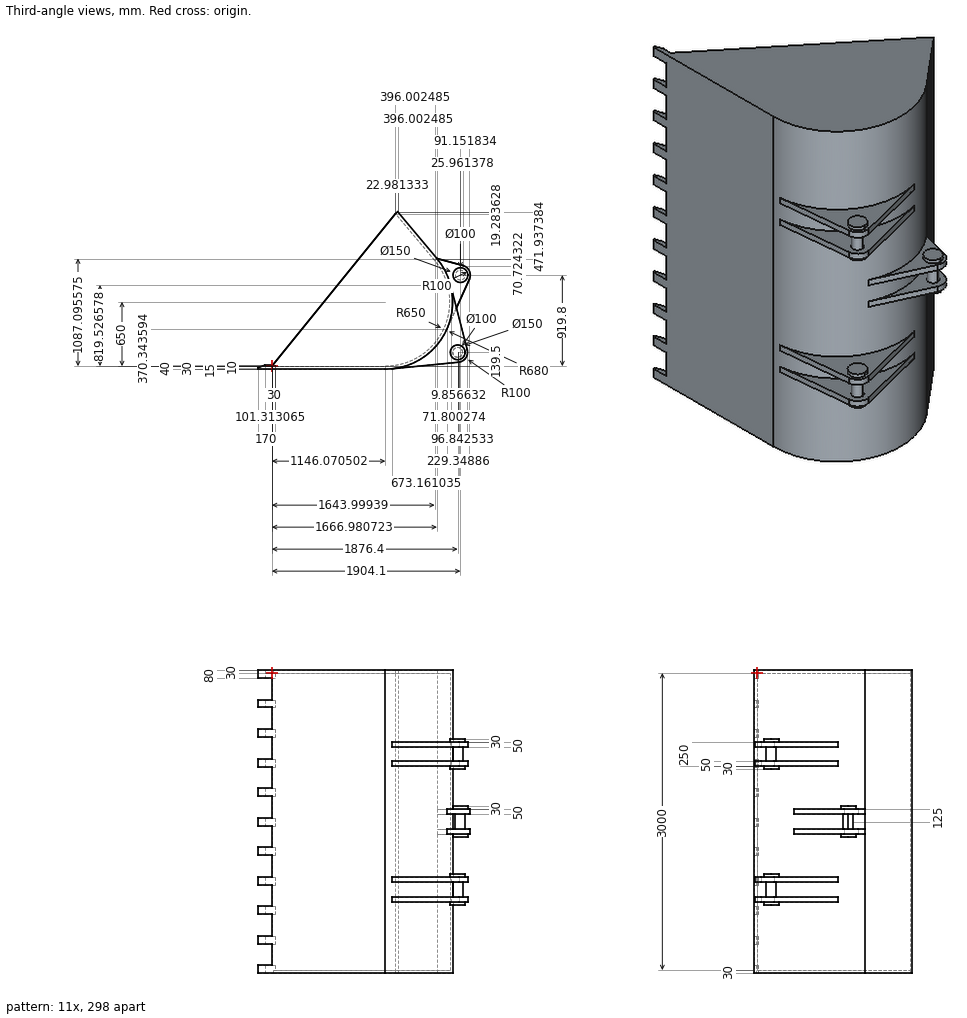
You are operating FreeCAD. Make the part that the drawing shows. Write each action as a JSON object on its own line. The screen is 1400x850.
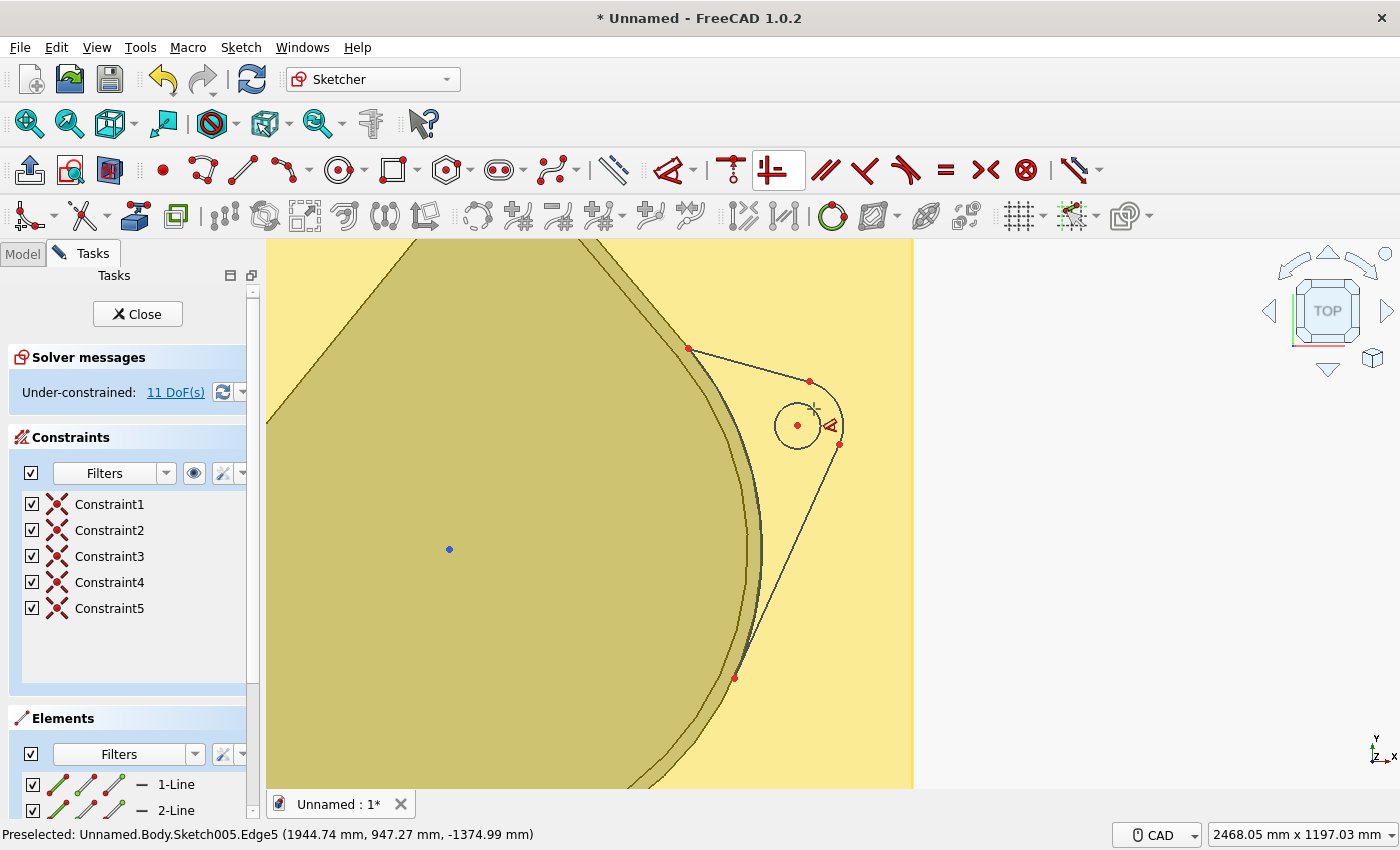
{"action": "left_click", "coordinate": [761, 578]}
{"action": "left_click", "coordinate": [793, 581]}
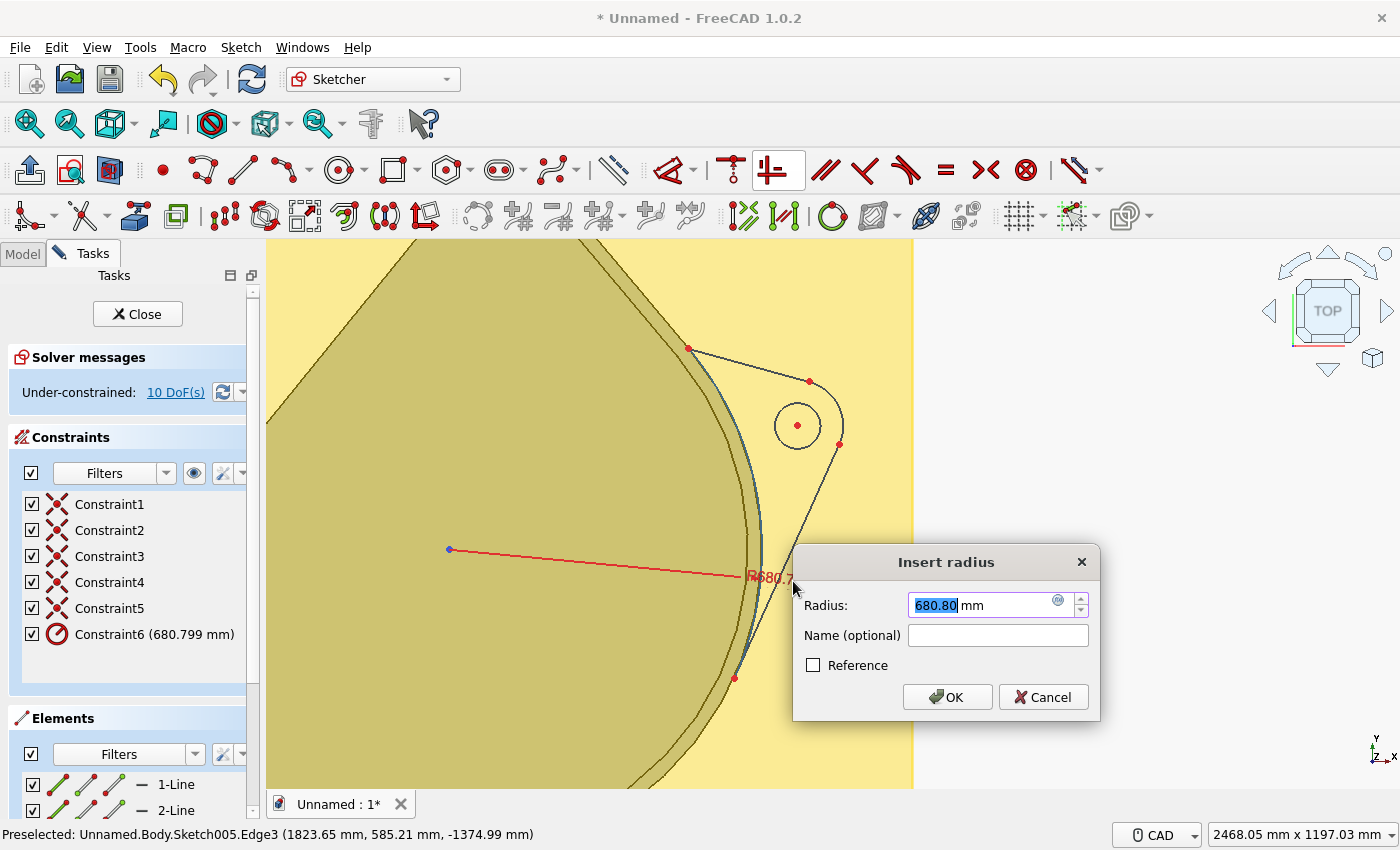
{"action": "type", "text": "680"}
{"action": "key", "text": "Return"}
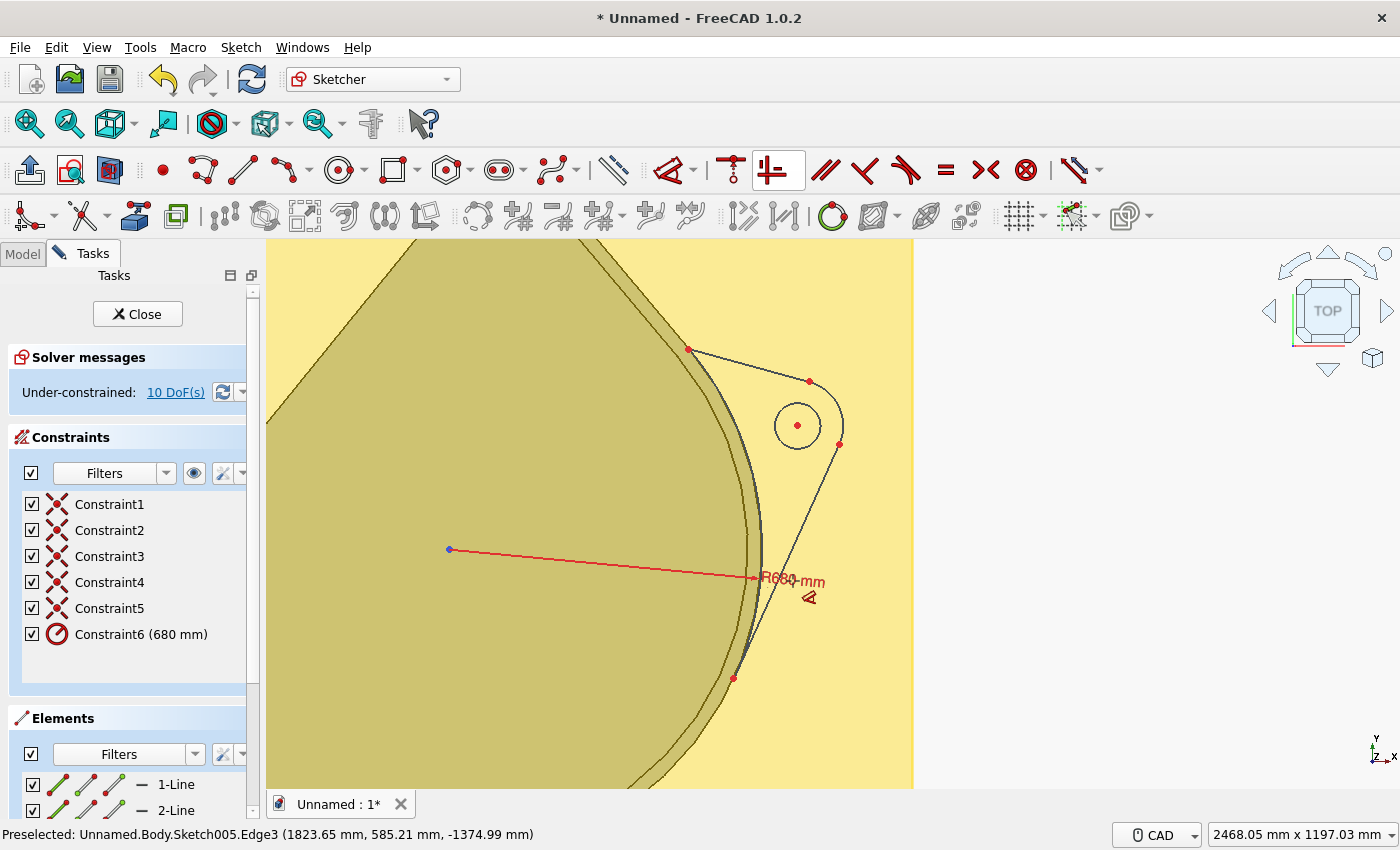
{"action": "left_click", "coordinate": [843, 422]}
{"action": "left_click", "coordinate": [875, 419]}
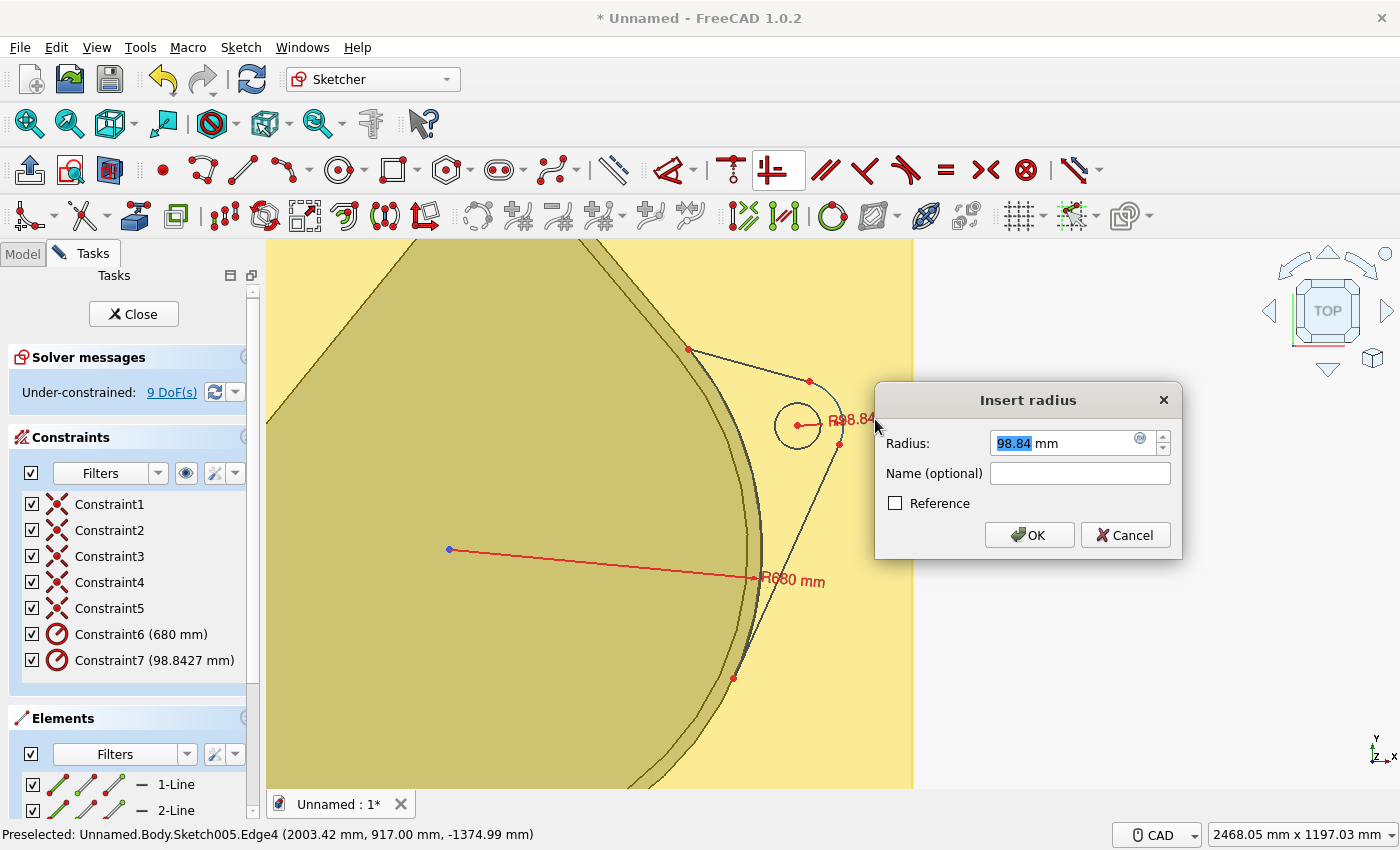
{"action": "type", "text": "100"}
{"action": "key", "text": "Return"}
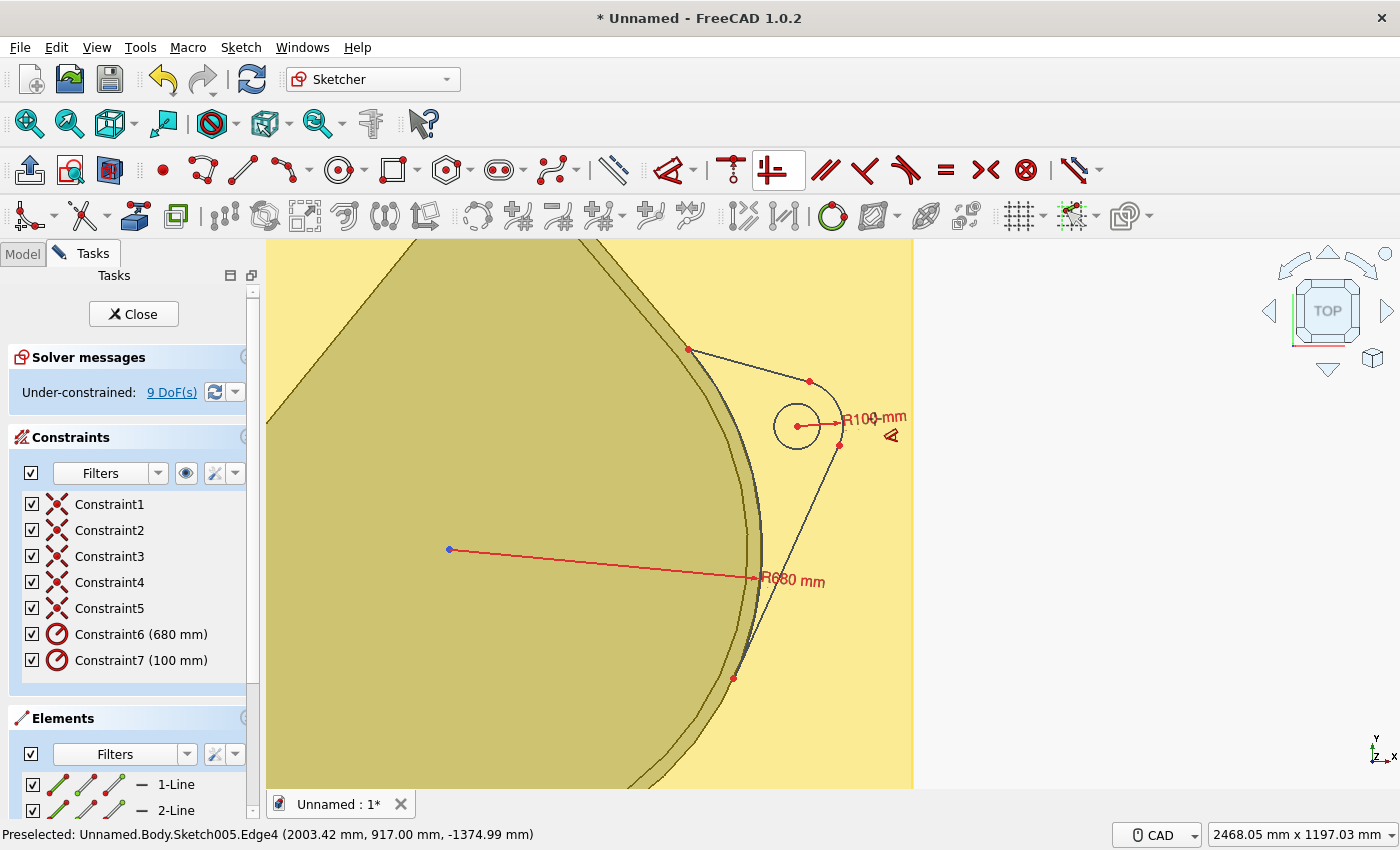
{"action": "left_click", "coordinate": [813, 410]}
{"action": "left_click", "coordinate": [758, 388]}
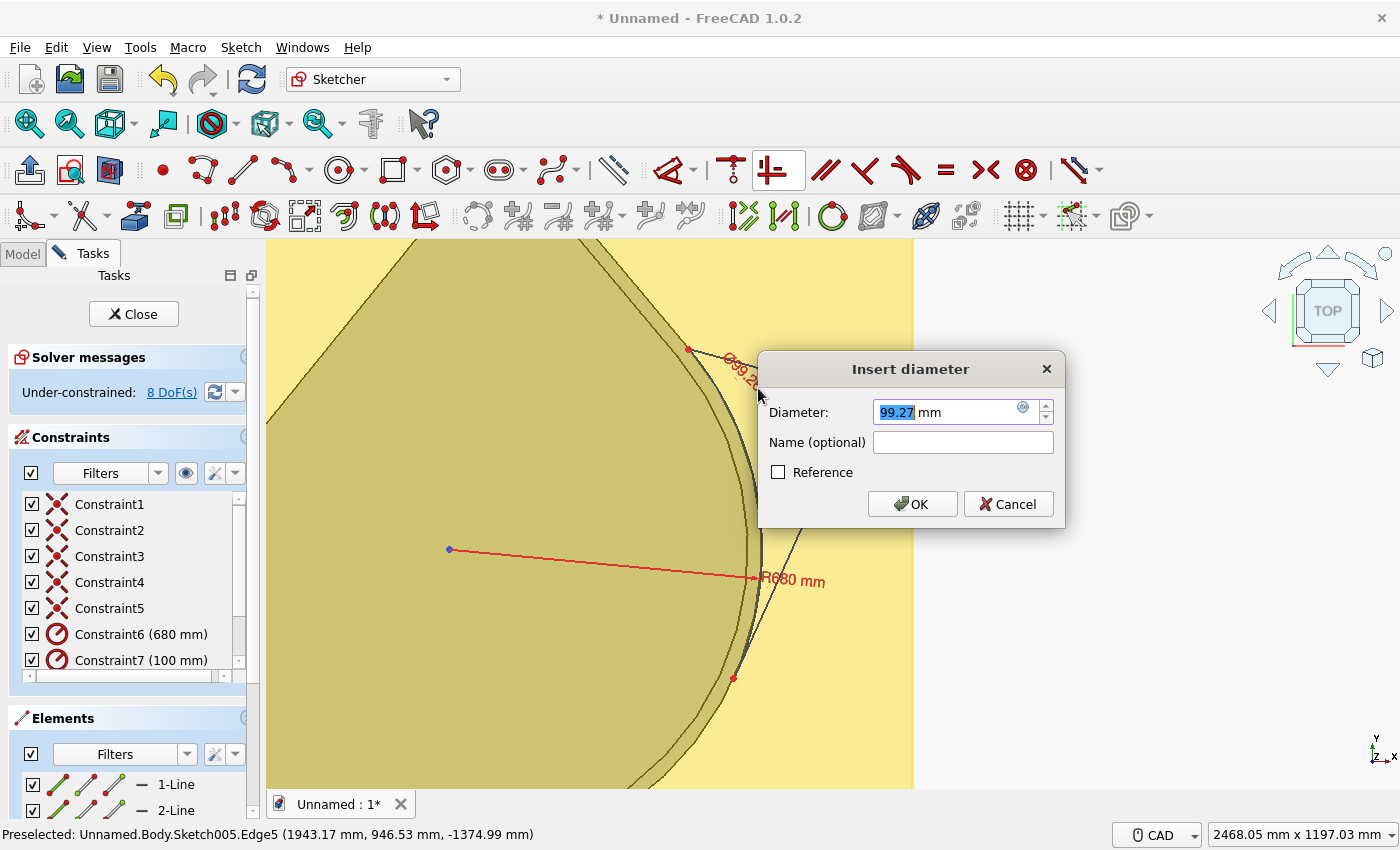
{"action": "type", "text": "100"}
{"action": "key", "text": "Return"}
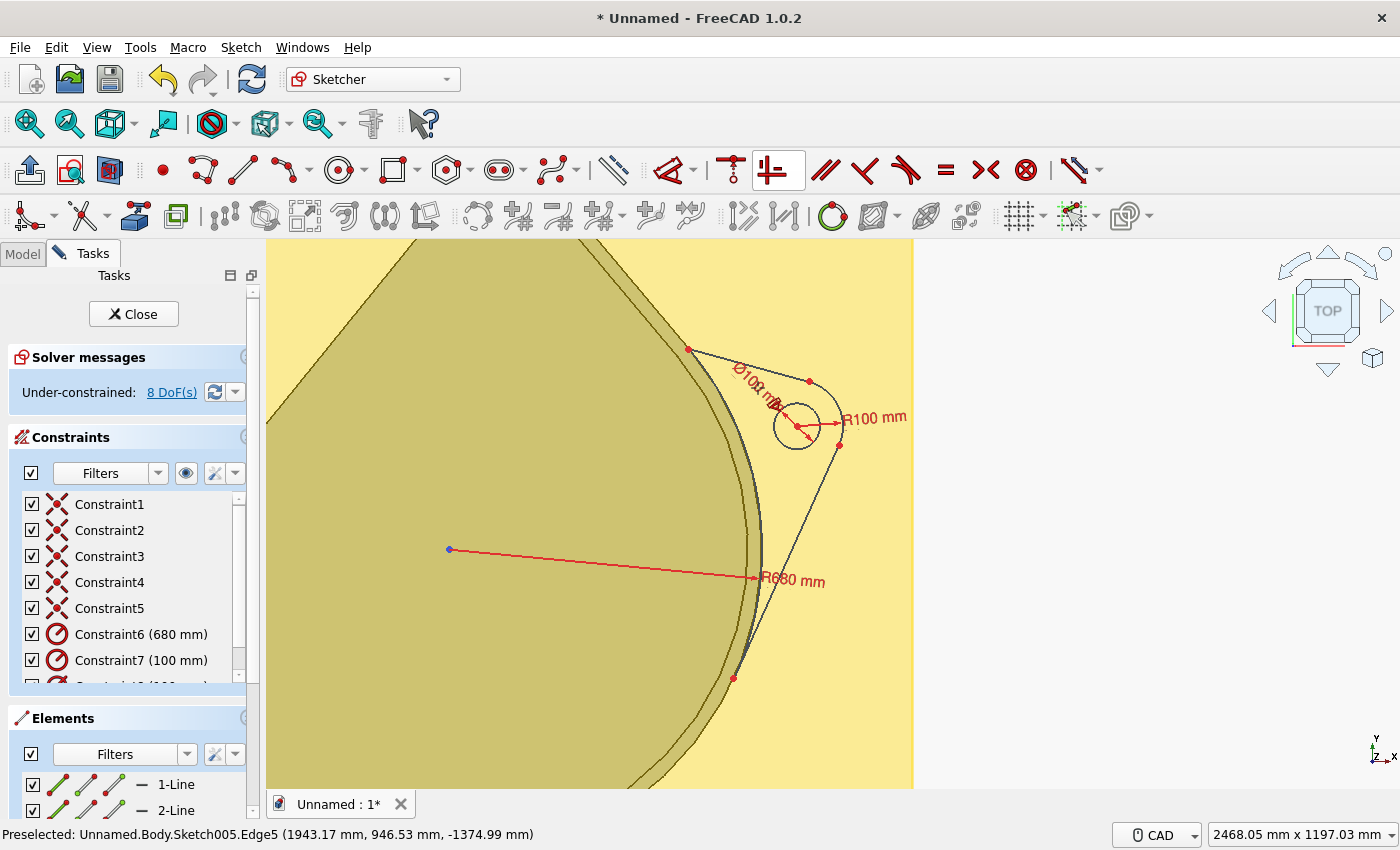
{"action": "left_click", "coordinate": [450, 550]}
{"action": "left_click", "coordinate": [484, 655]}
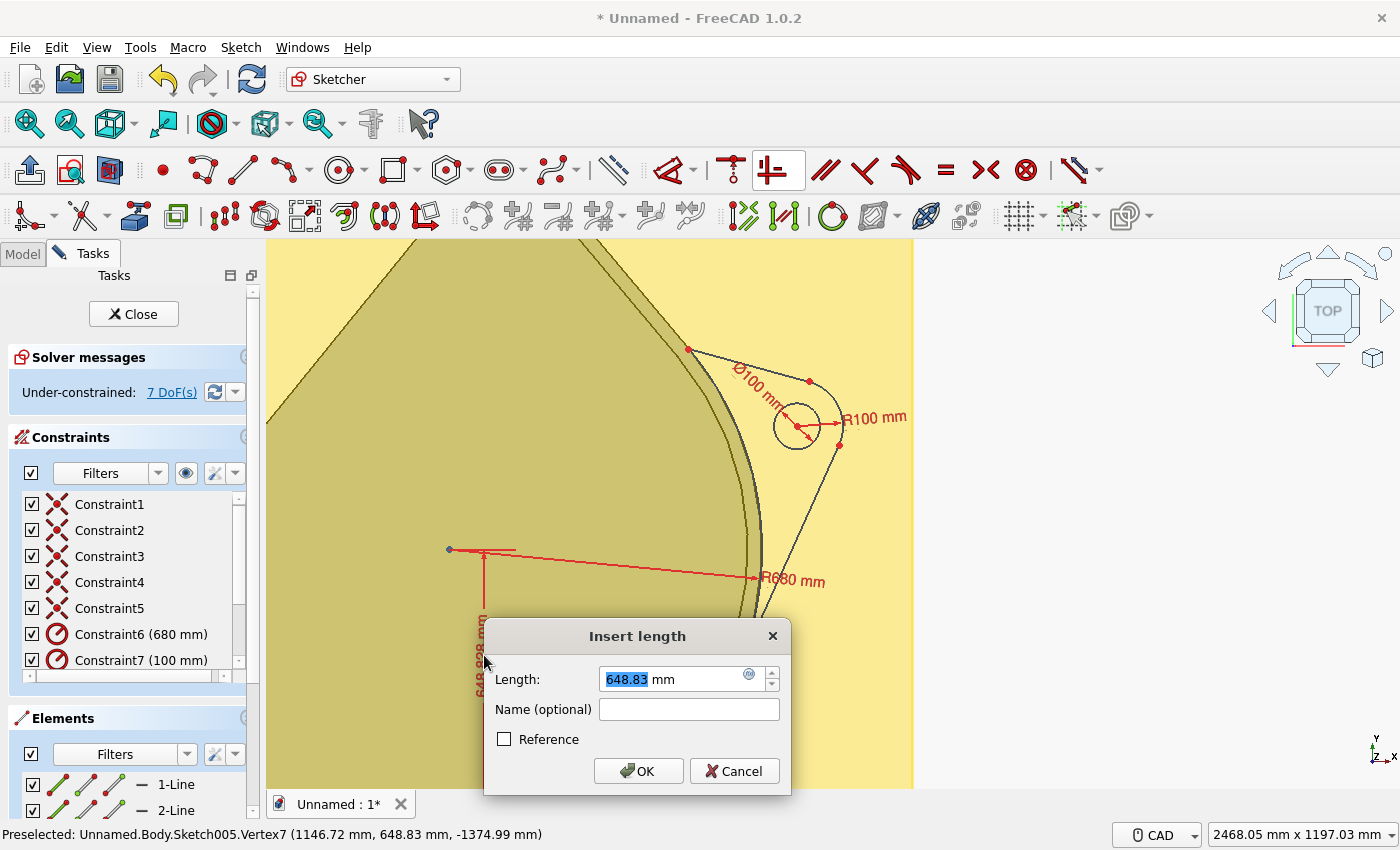
{"action": "type", "text": "650"}
{"action": "key", "text": "Return"}